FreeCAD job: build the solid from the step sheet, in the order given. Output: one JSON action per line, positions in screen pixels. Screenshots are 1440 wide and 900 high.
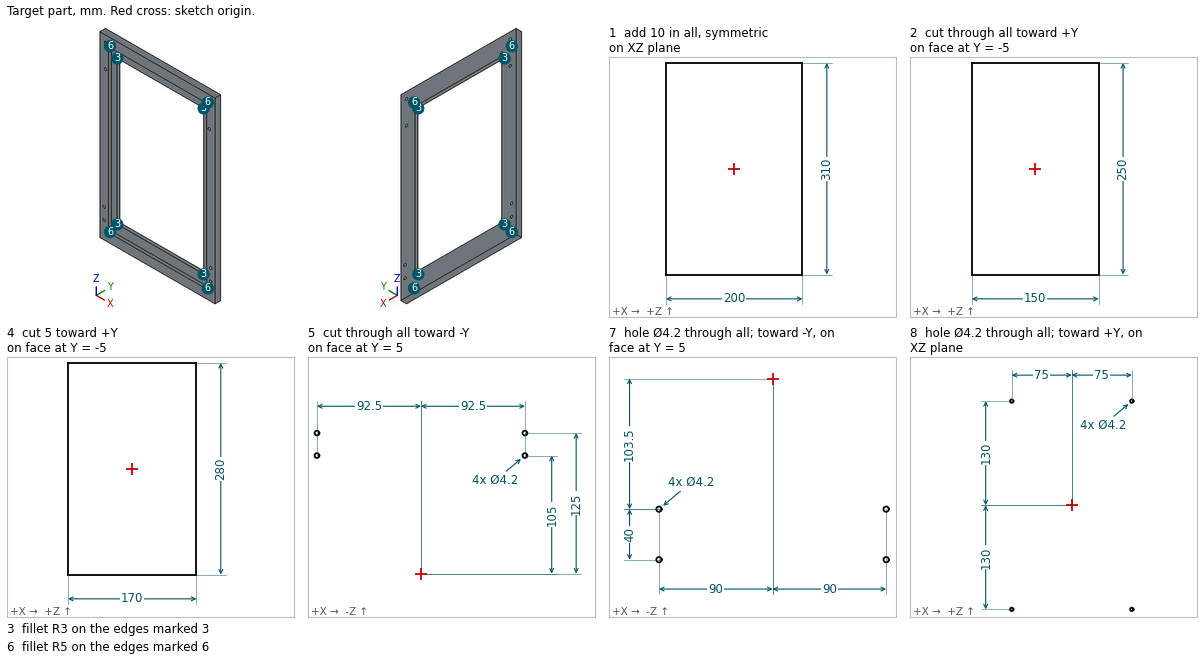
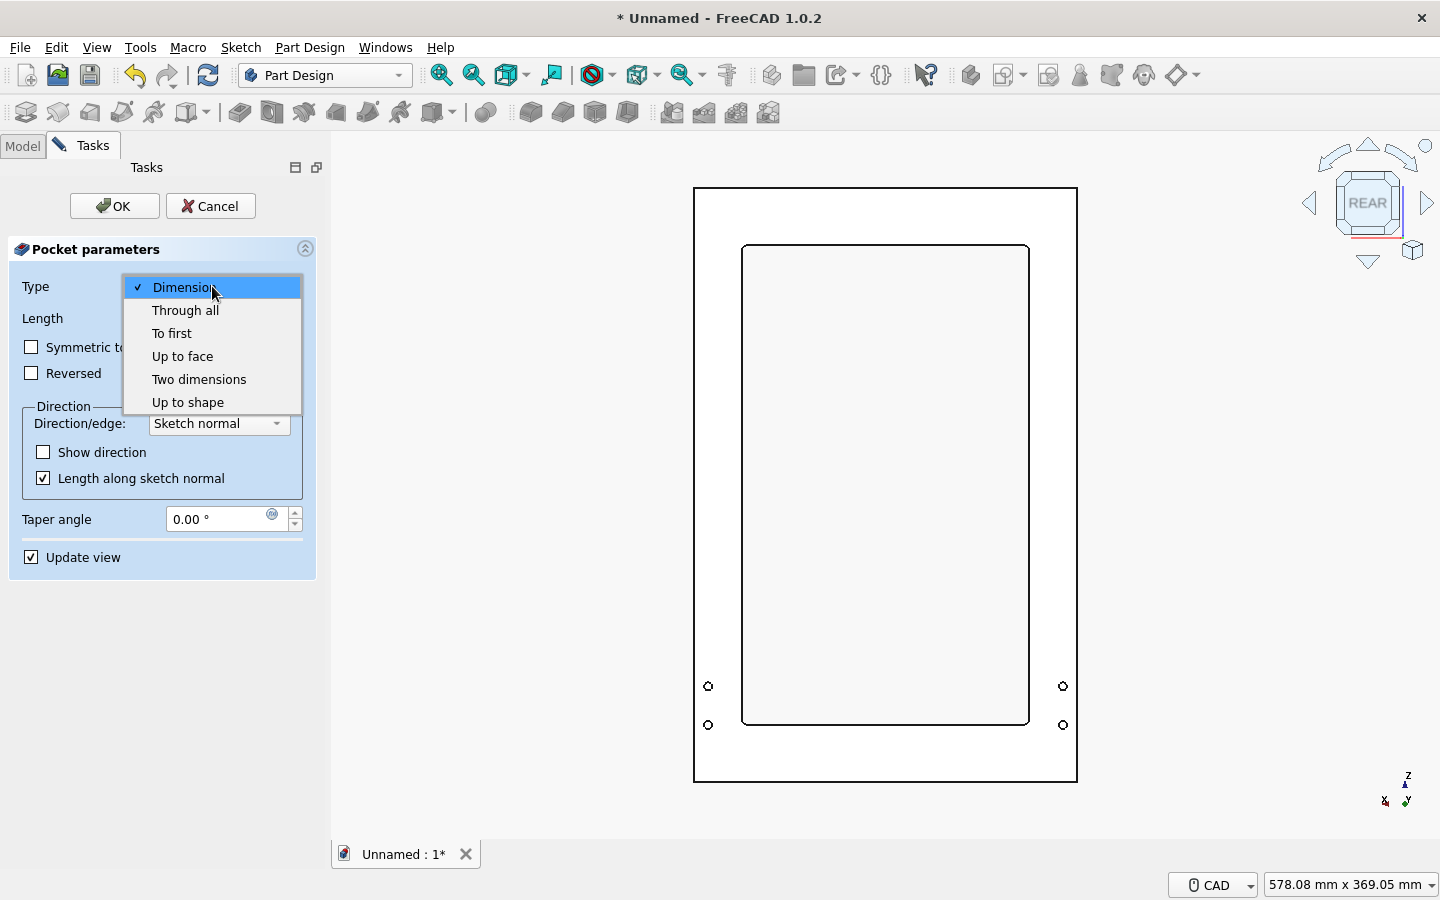
{"action": "left_click", "coordinate": [212, 310]}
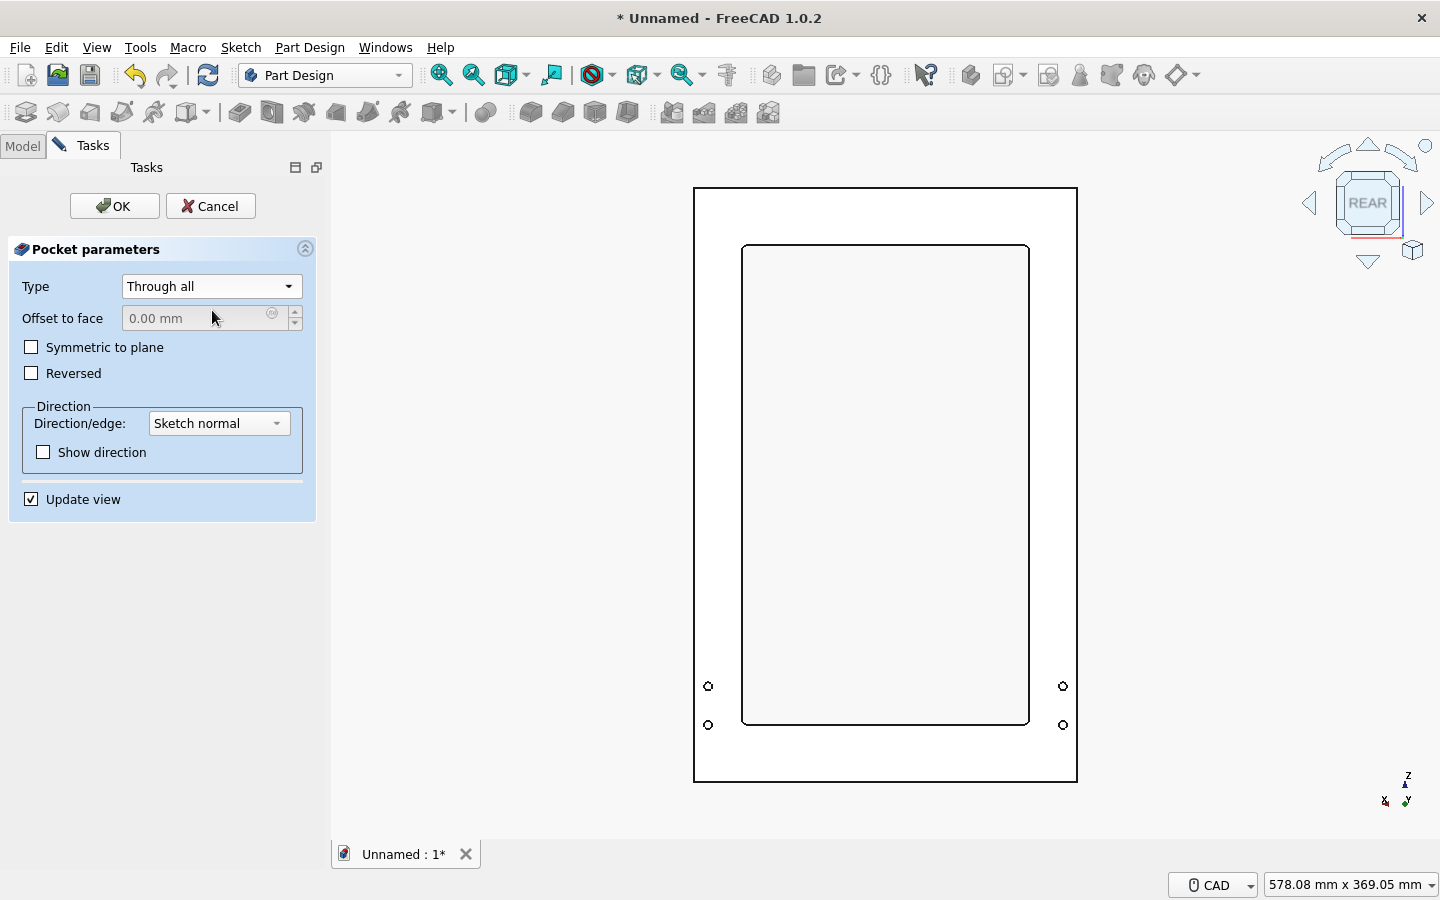
{"action": "left_click", "coordinate": [115, 206]}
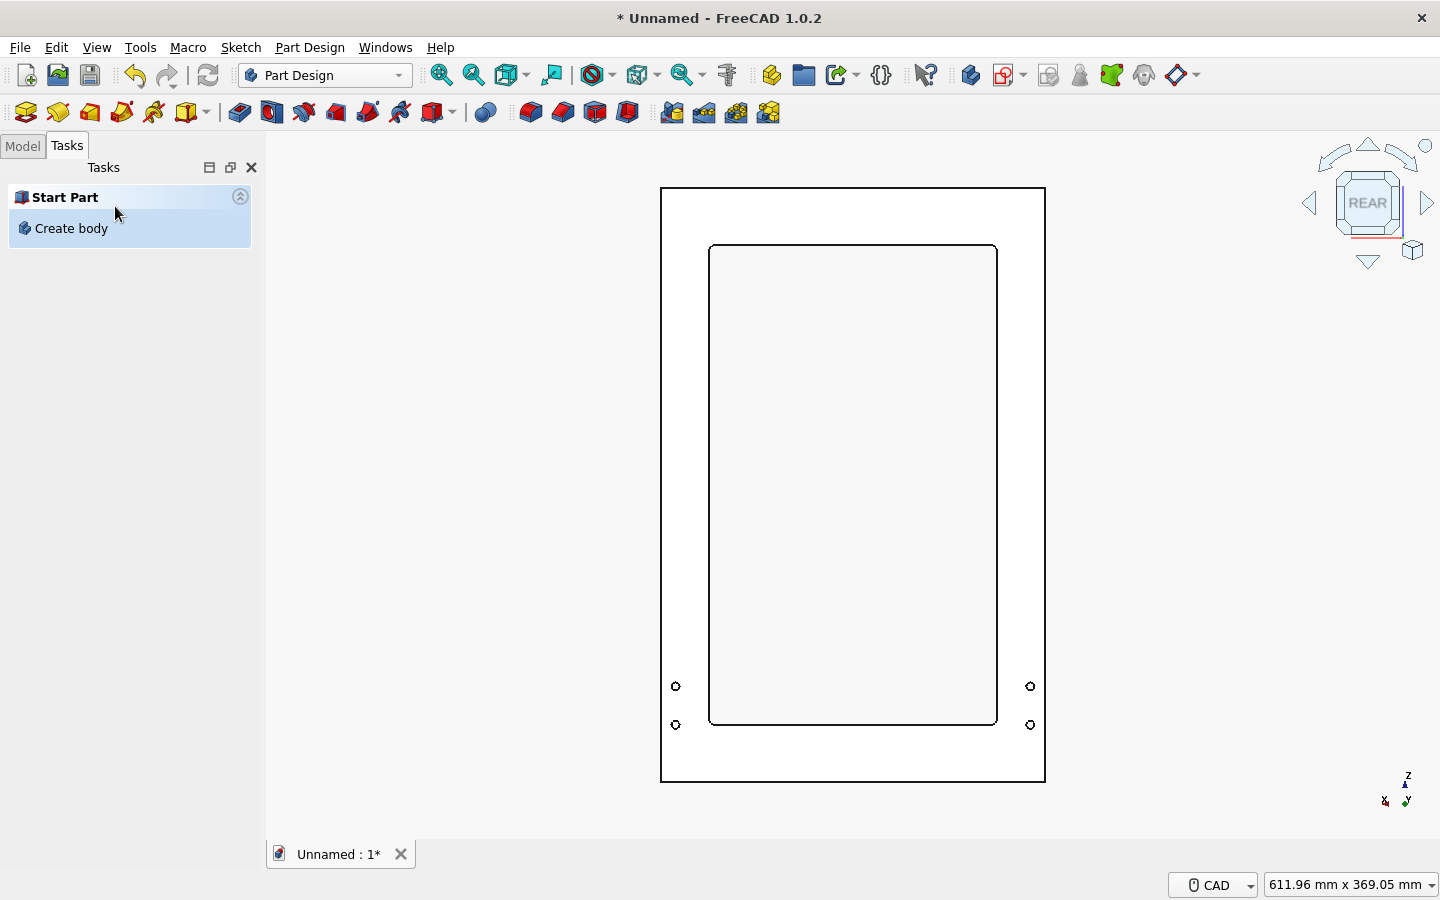
{"action": "scroll", "coordinate": [690, 215], "scroll_direction": "up", "scroll_amount": 8}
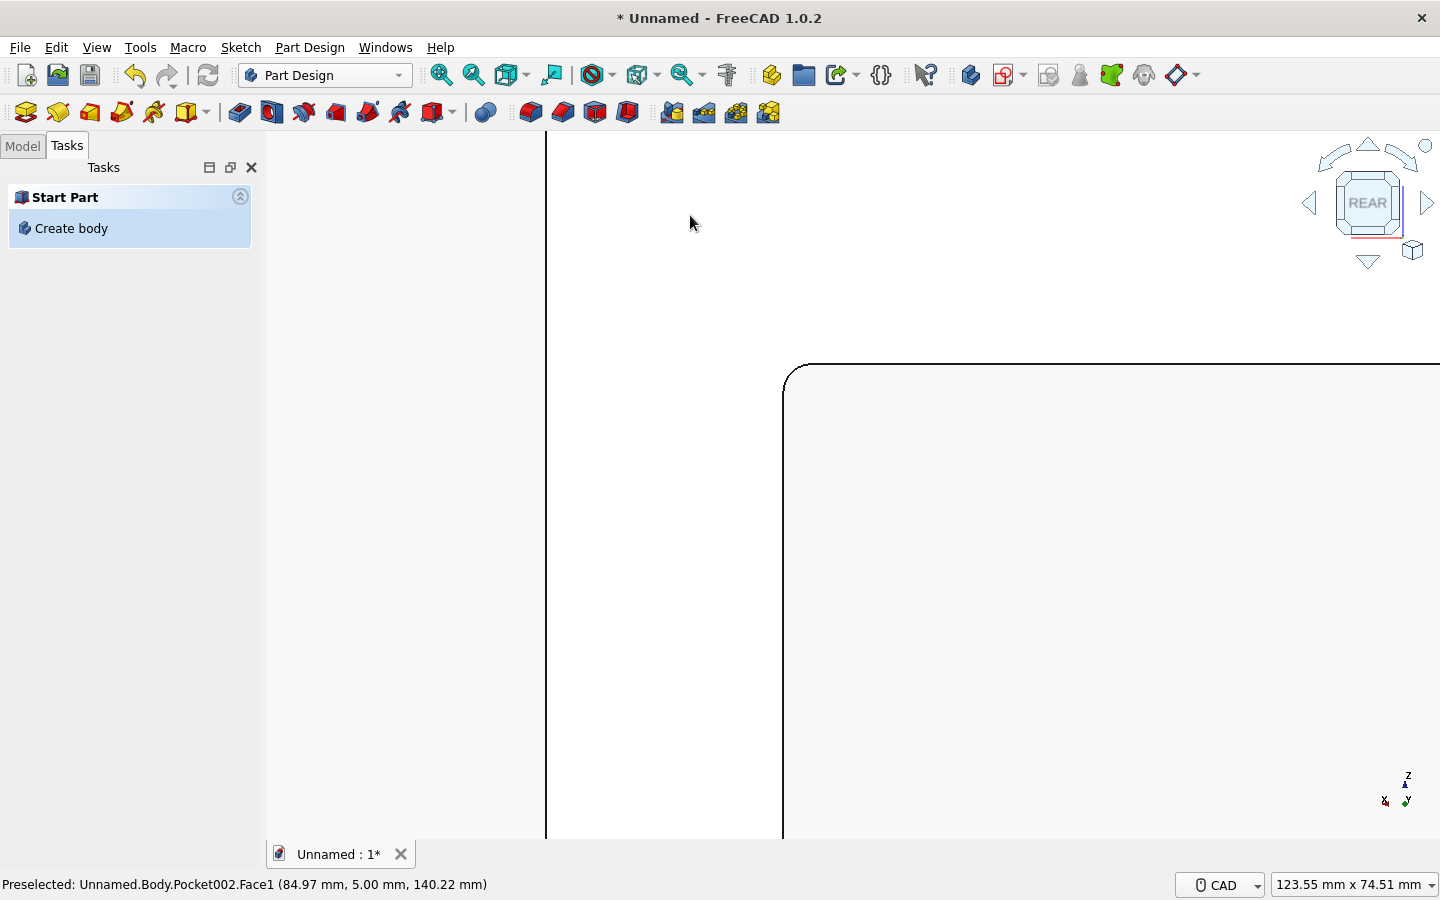
{"action": "key", "text": "v f"}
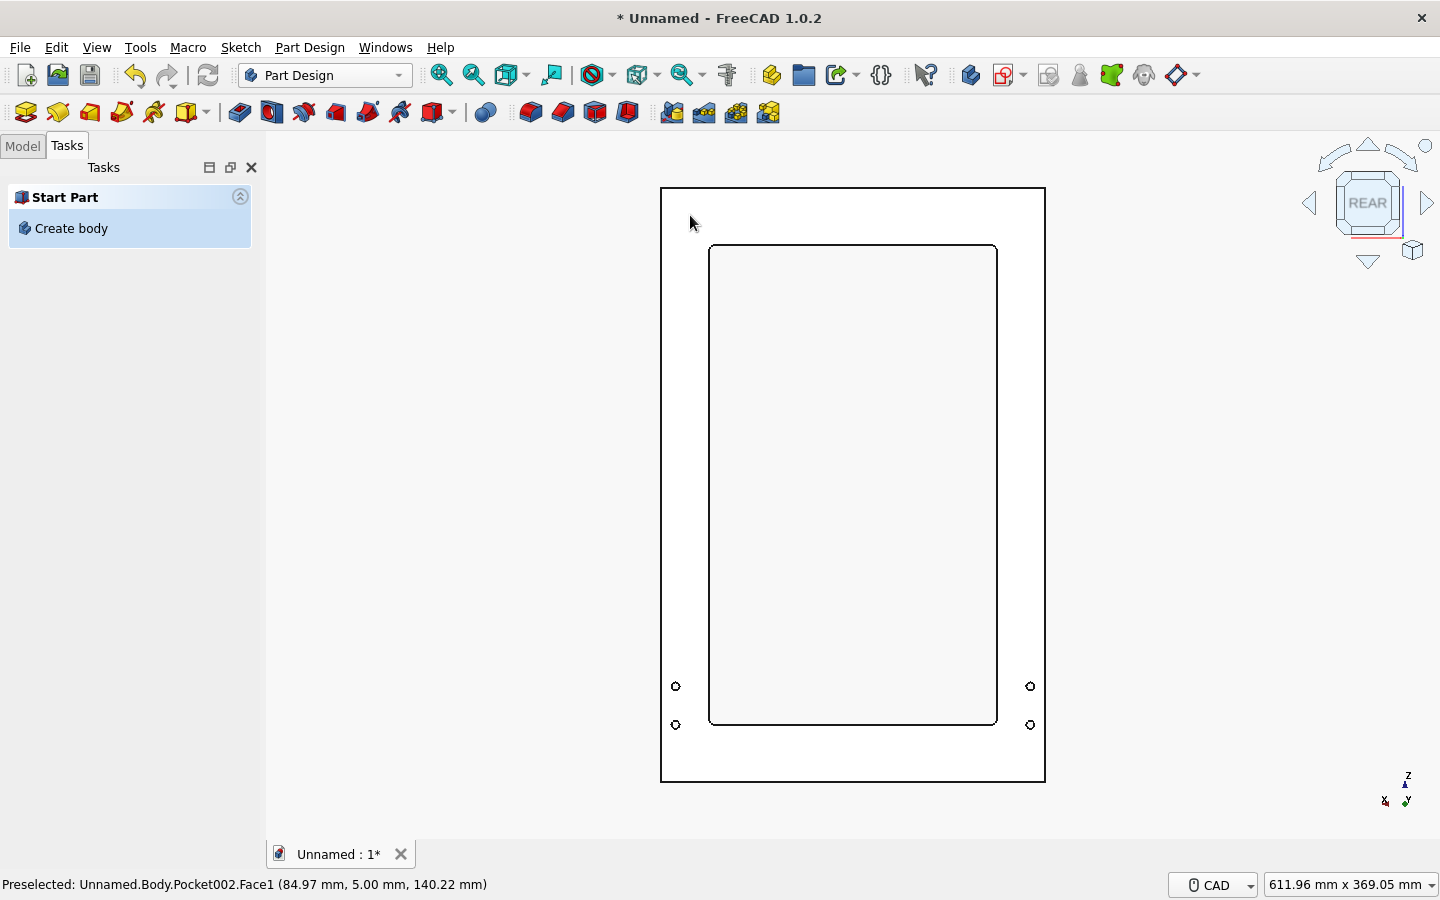
{"action": "key", "text": "0"}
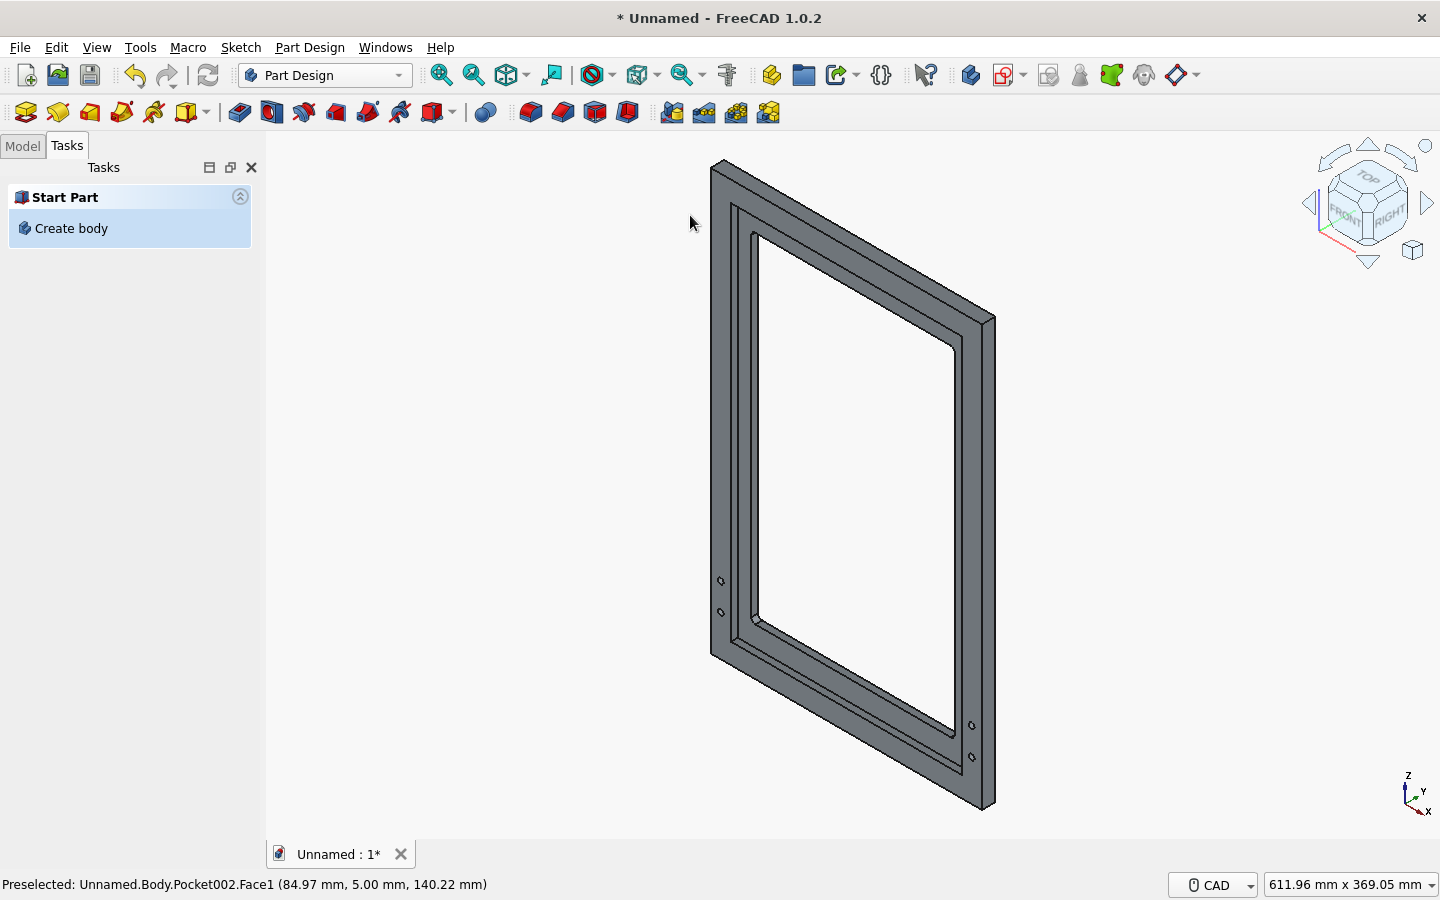
{"action": "scroll", "coordinate": [965, 333], "scroll_direction": "up", "scroll_amount": 8}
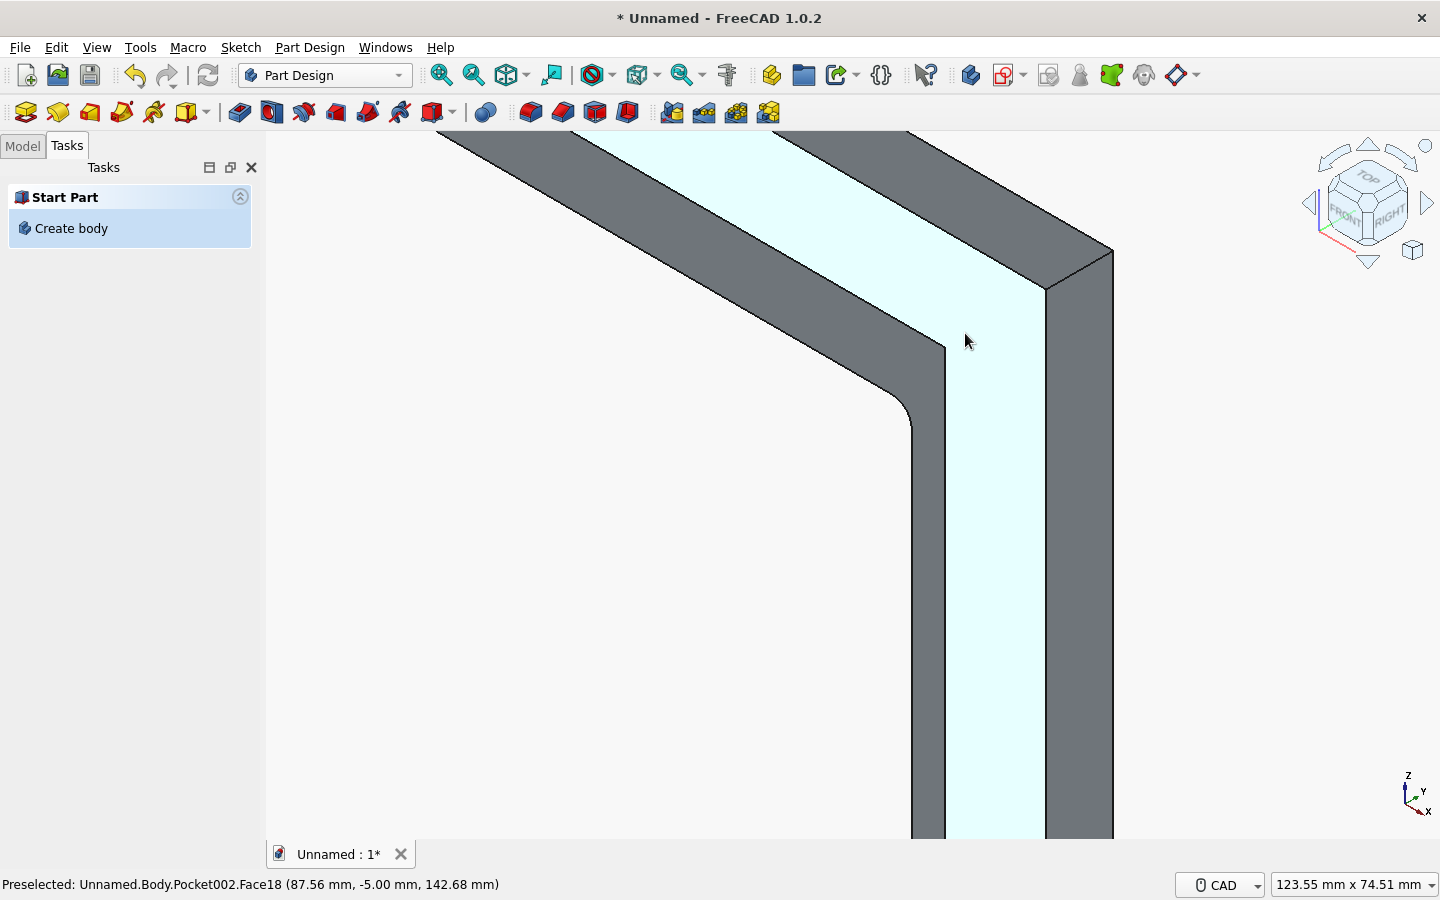
{"action": "key", "text": "v f"}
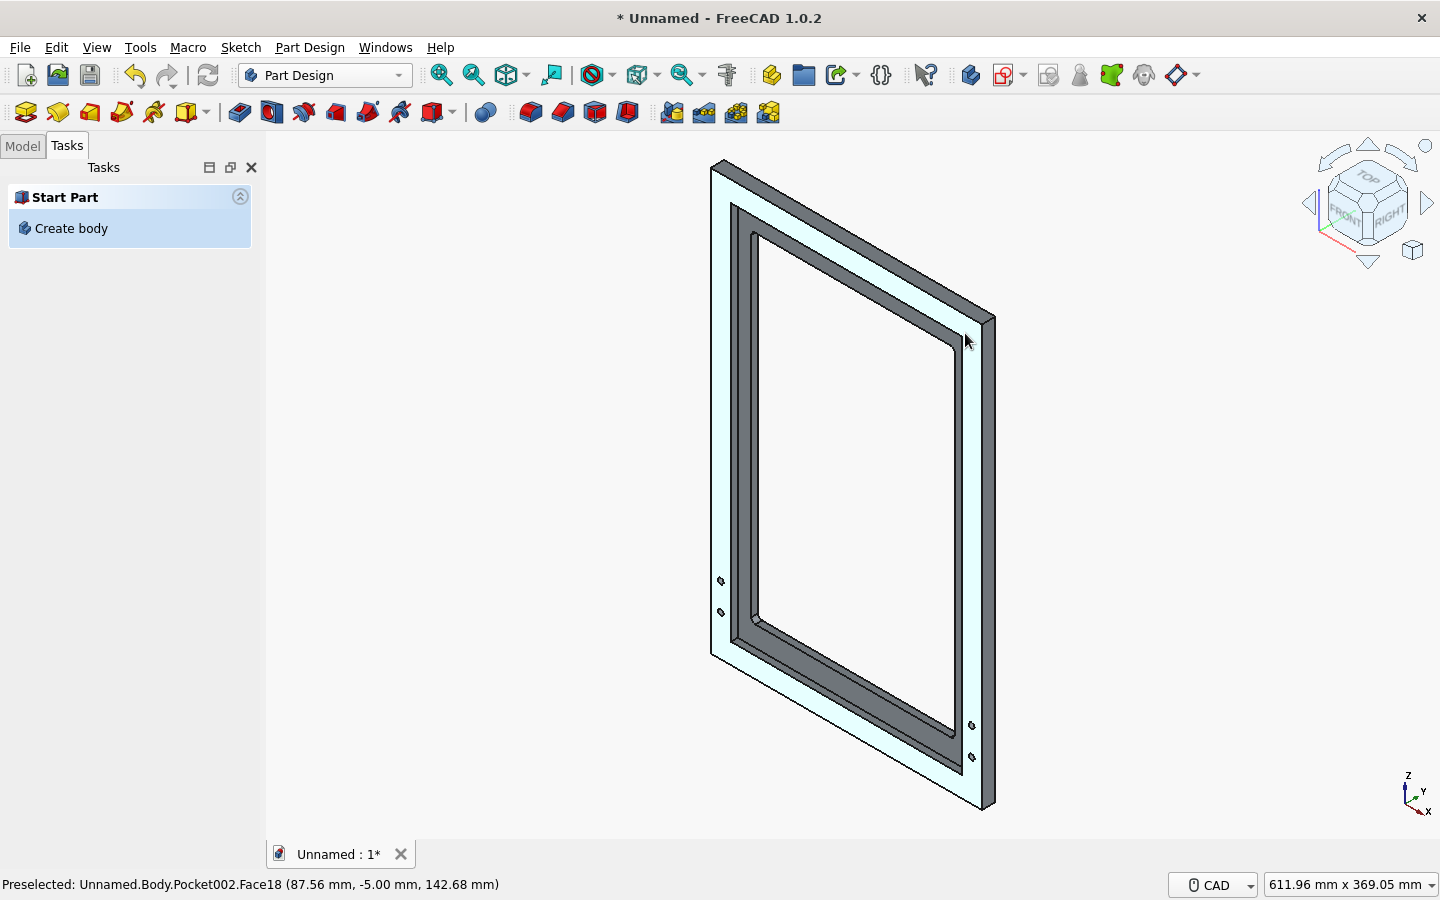
{"action": "key", "text": "2"}